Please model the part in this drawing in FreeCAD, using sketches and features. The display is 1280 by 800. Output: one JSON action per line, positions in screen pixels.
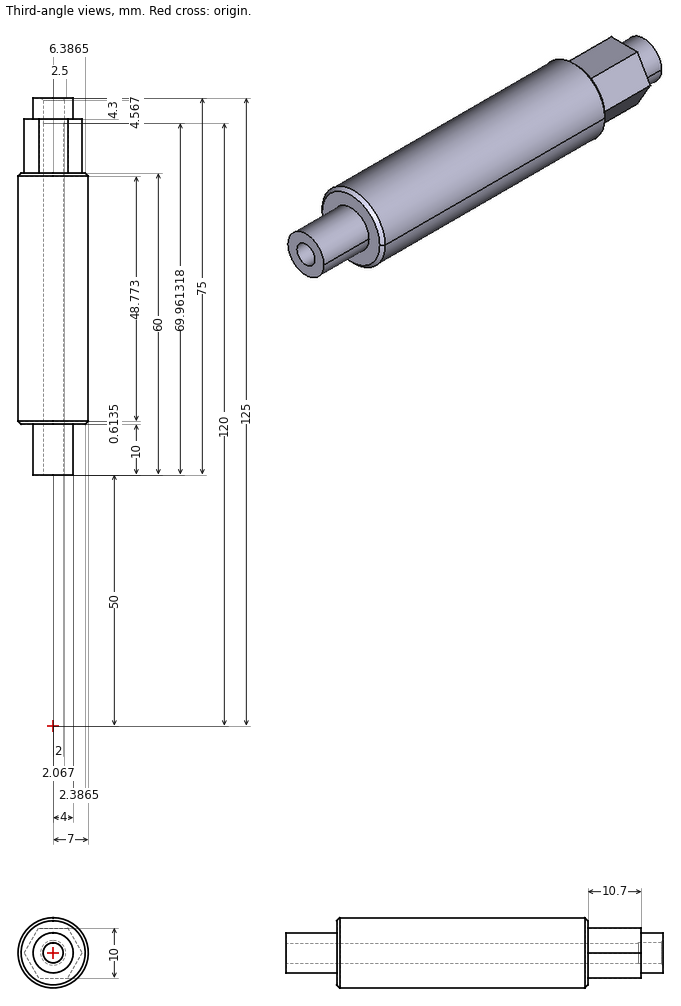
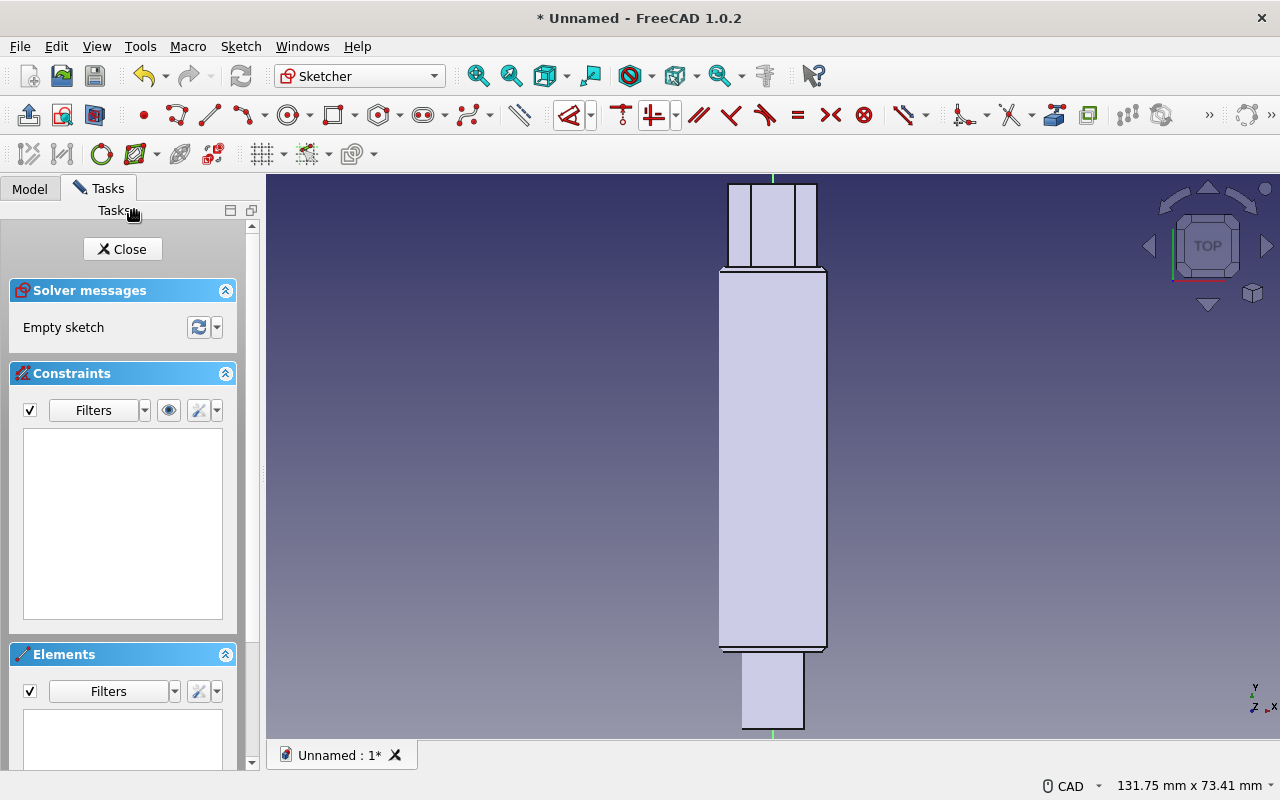
{"action": "left_click", "coordinate": [95, 116]}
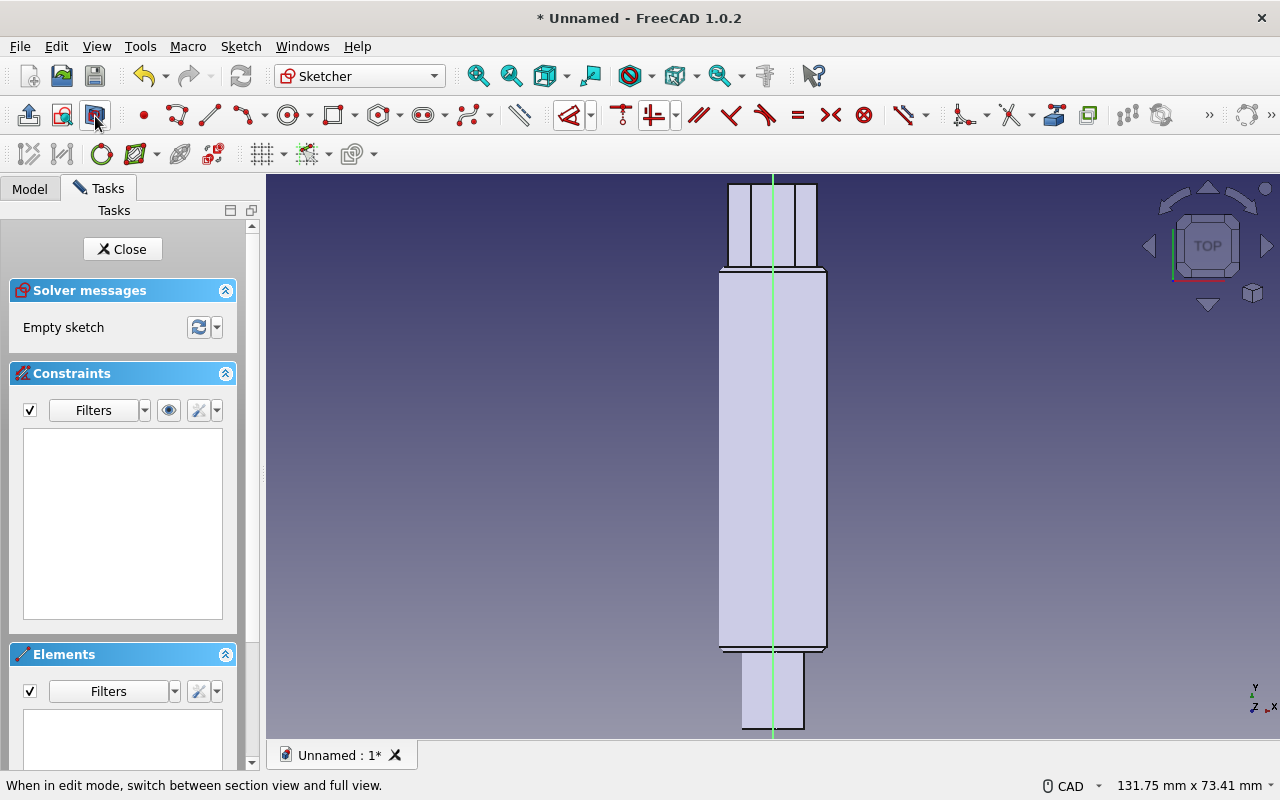
{"action": "scroll", "coordinate": [704, 456], "scroll_direction": "down", "scroll_amount": 5}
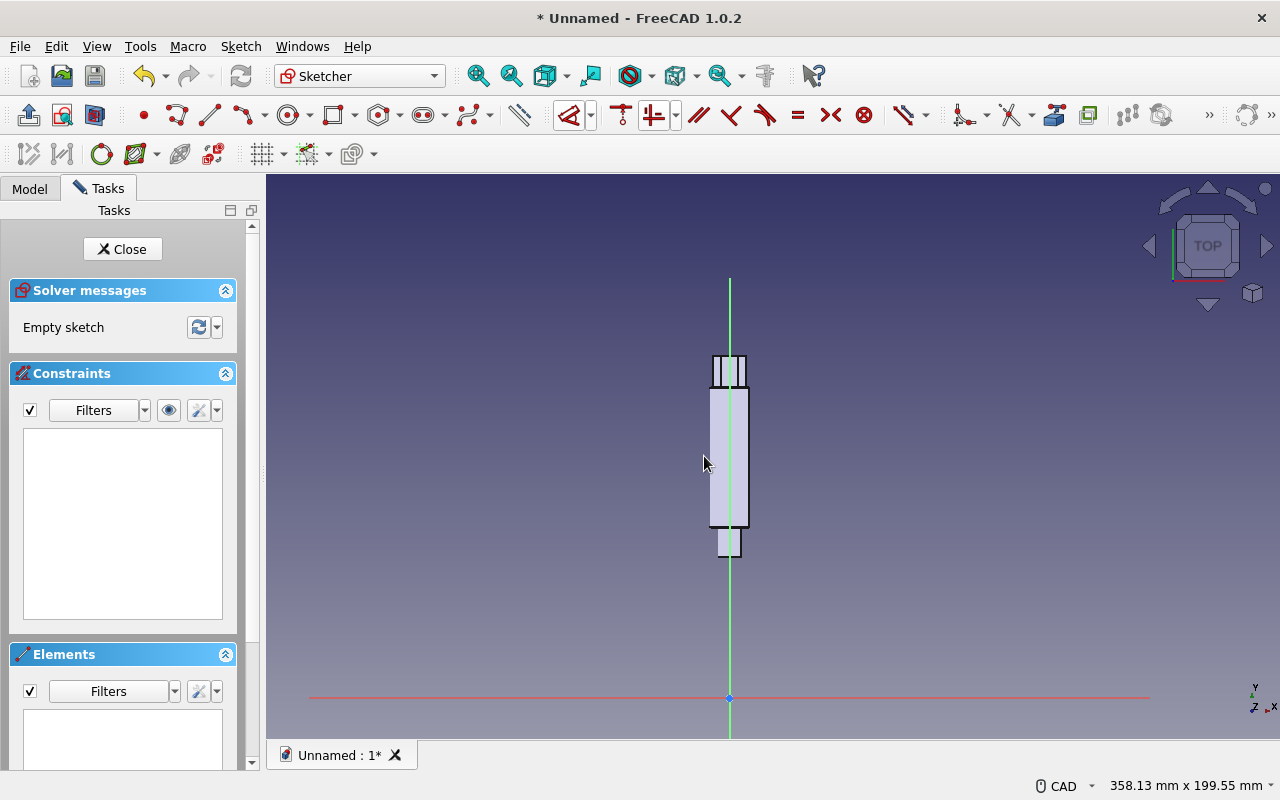
{"action": "scroll", "coordinate": [737, 345], "scroll_direction": "up", "scroll_amount": 15}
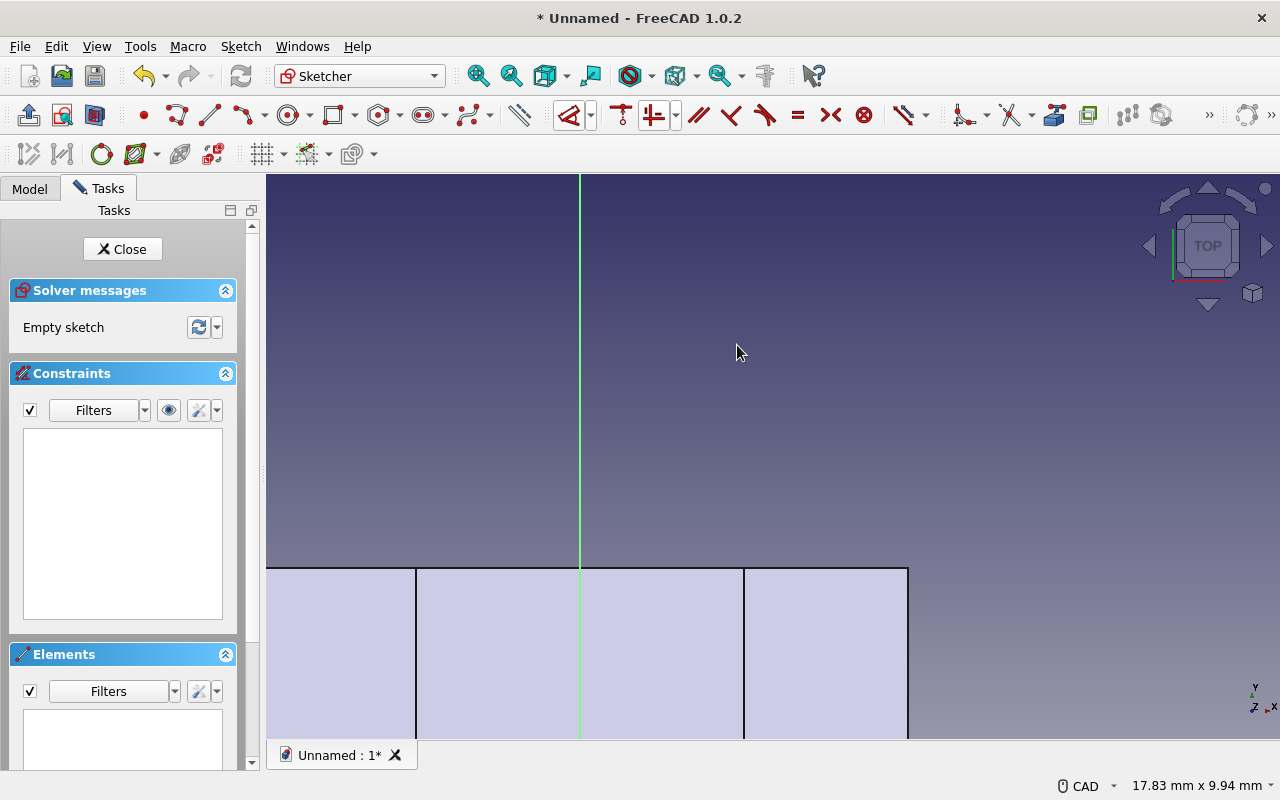
{"action": "scroll", "coordinate": [671, 425], "scroll_direction": "up", "scroll_amount": 2}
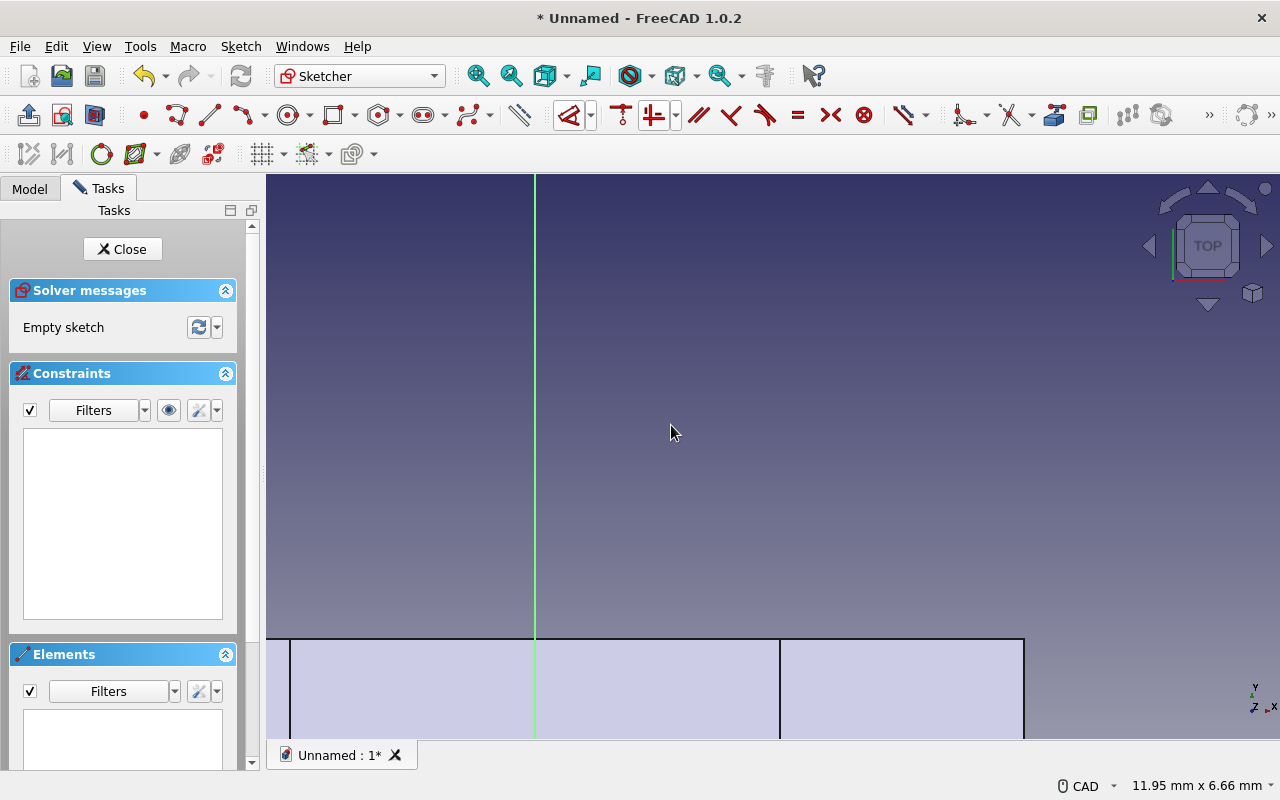
{"action": "left_click", "coordinate": [332, 116]}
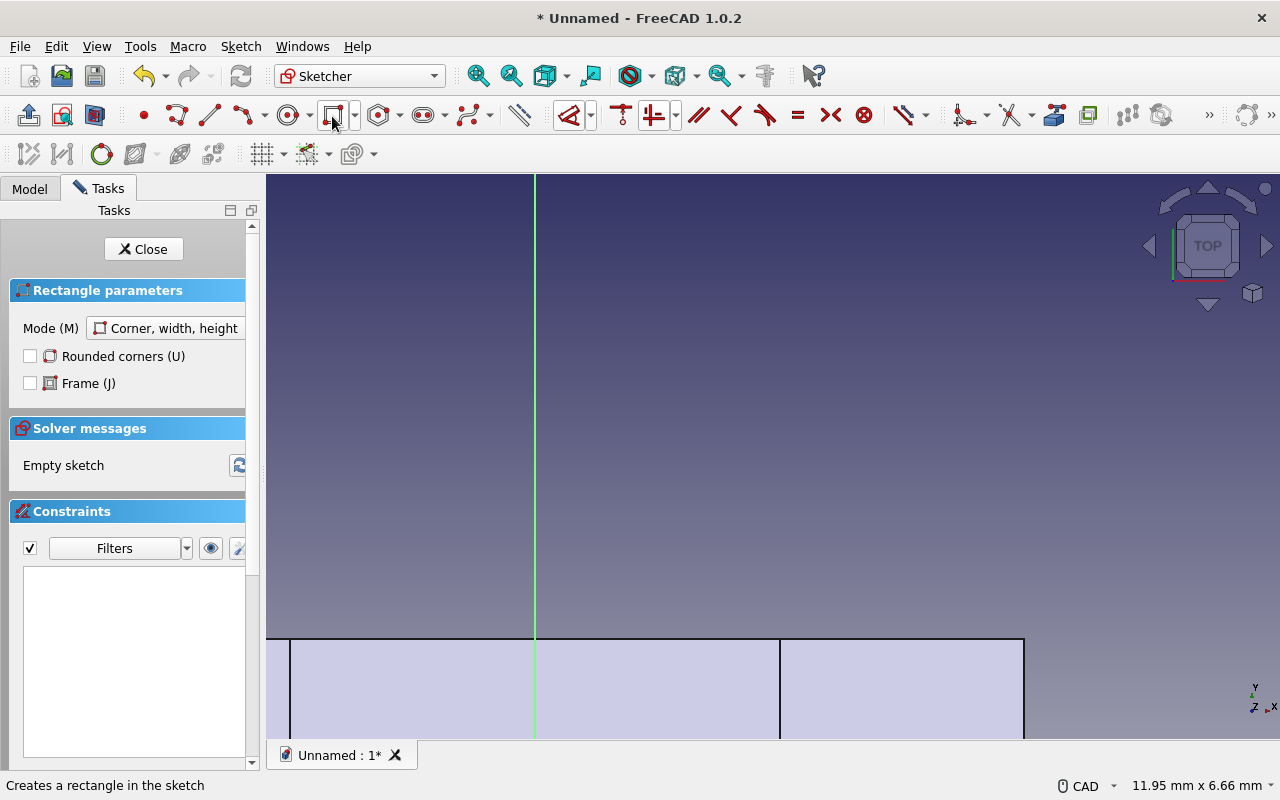
{"action": "left_click", "coordinate": [535, 274]}
{"action": "mouse_move", "coordinate": [874, 639]}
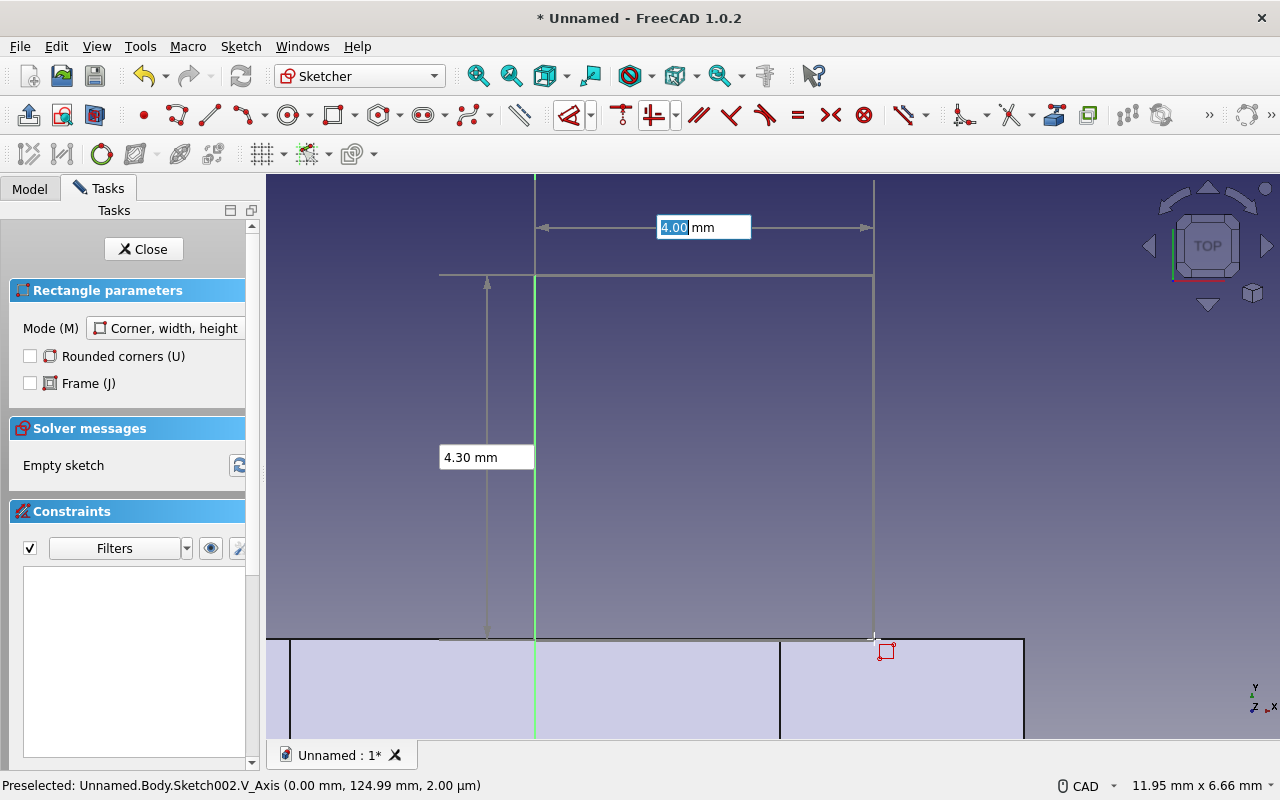
{"action": "type", "text": "4"}
{"action": "key", "text": "Tab"}
{"action": "type", "text": "4.3"}
{"action": "key", "text": "Return"}
{"action": "key", "text": "Escape"}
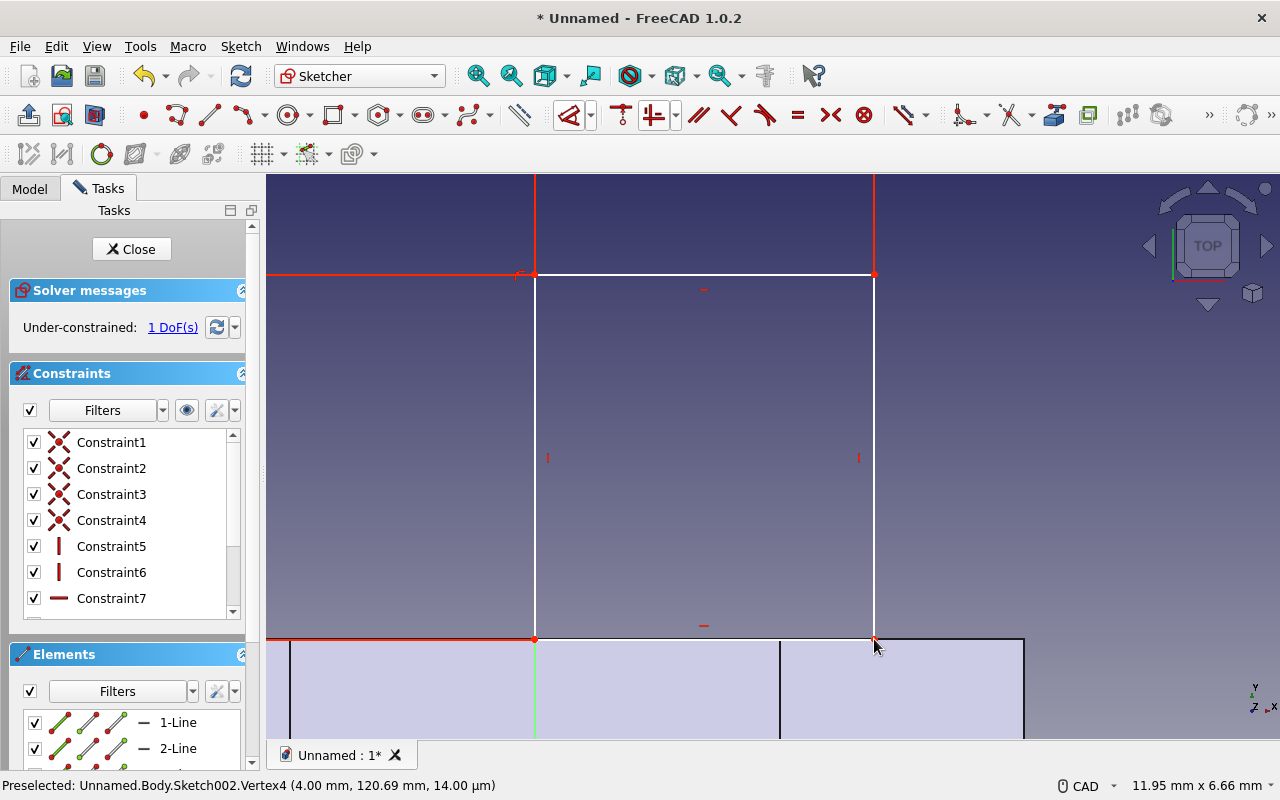
{"action": "left_click", "coordinate": [535, 275]}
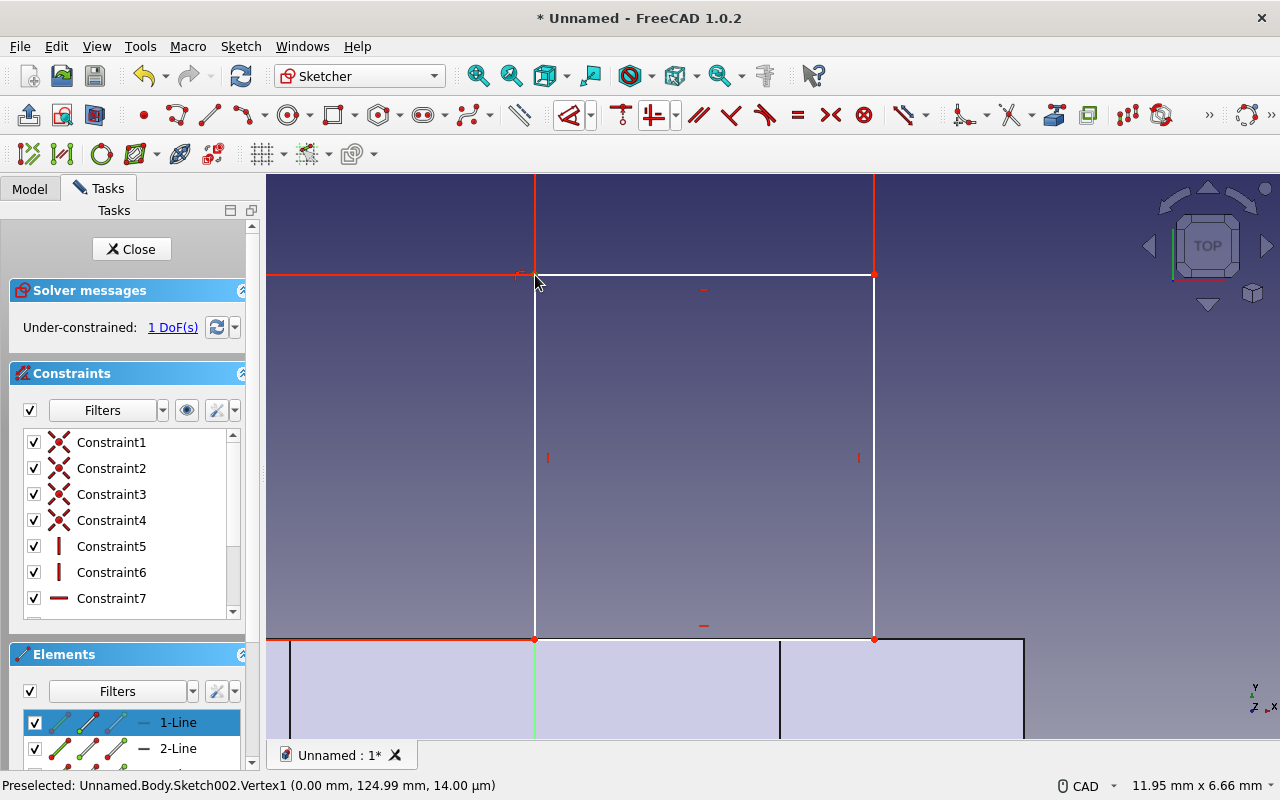
{"action": "left_click", "coordinate": [590, 116]}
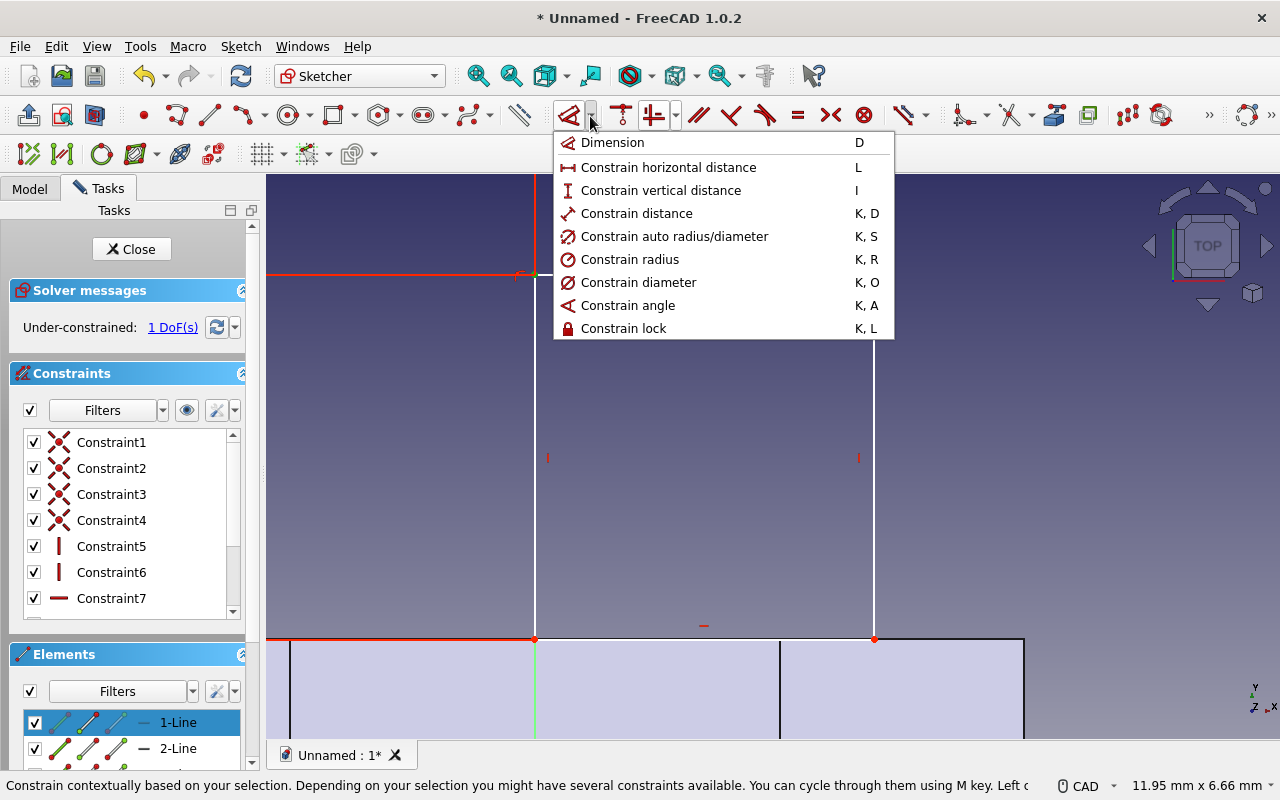
{"action": "left_click", "coordinate": [724, 190]}